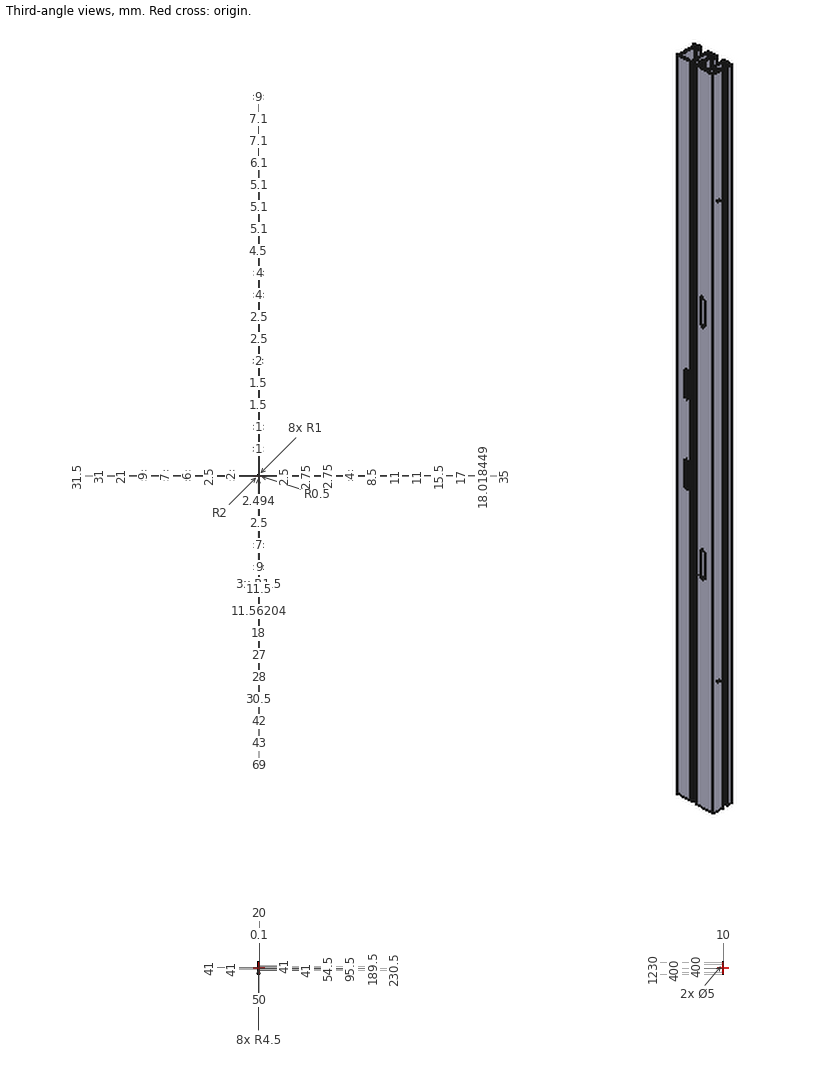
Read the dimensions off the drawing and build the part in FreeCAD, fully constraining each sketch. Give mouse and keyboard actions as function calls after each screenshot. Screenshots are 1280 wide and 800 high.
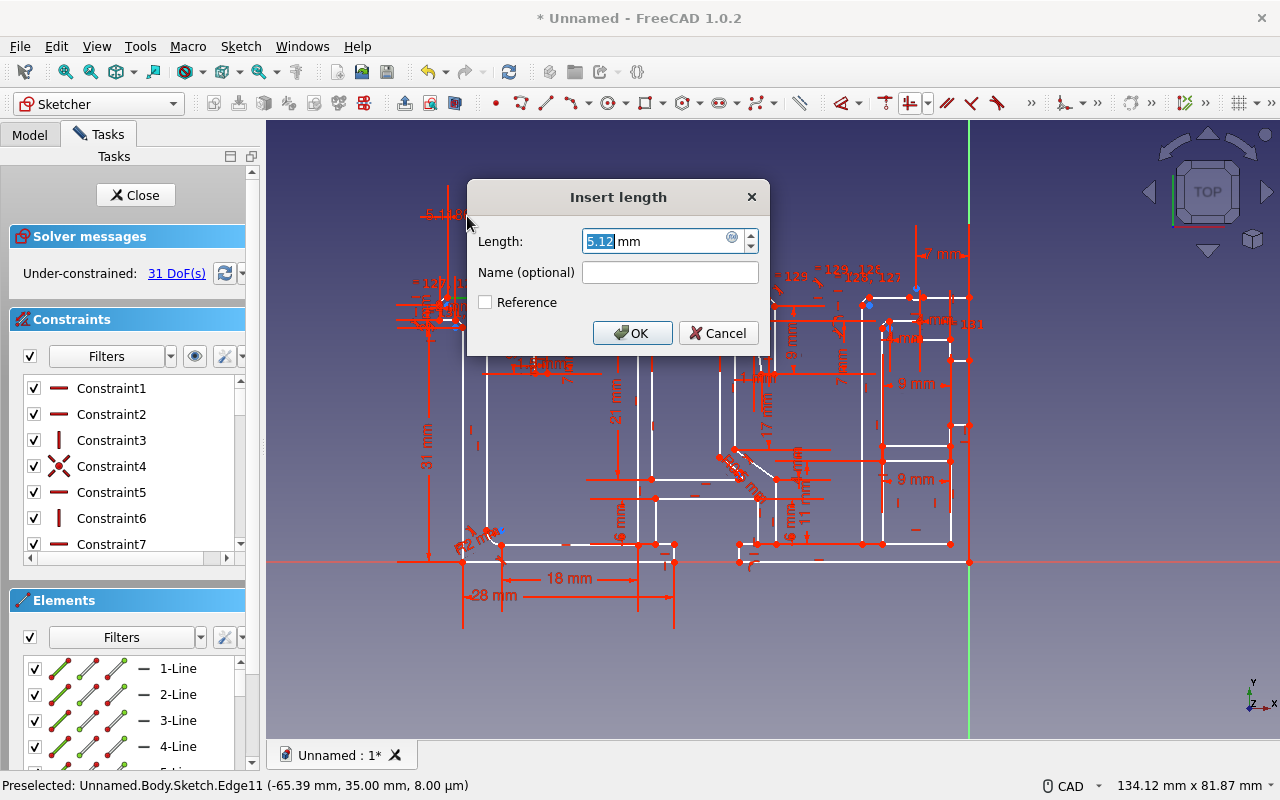
text(5.1)
key(Return)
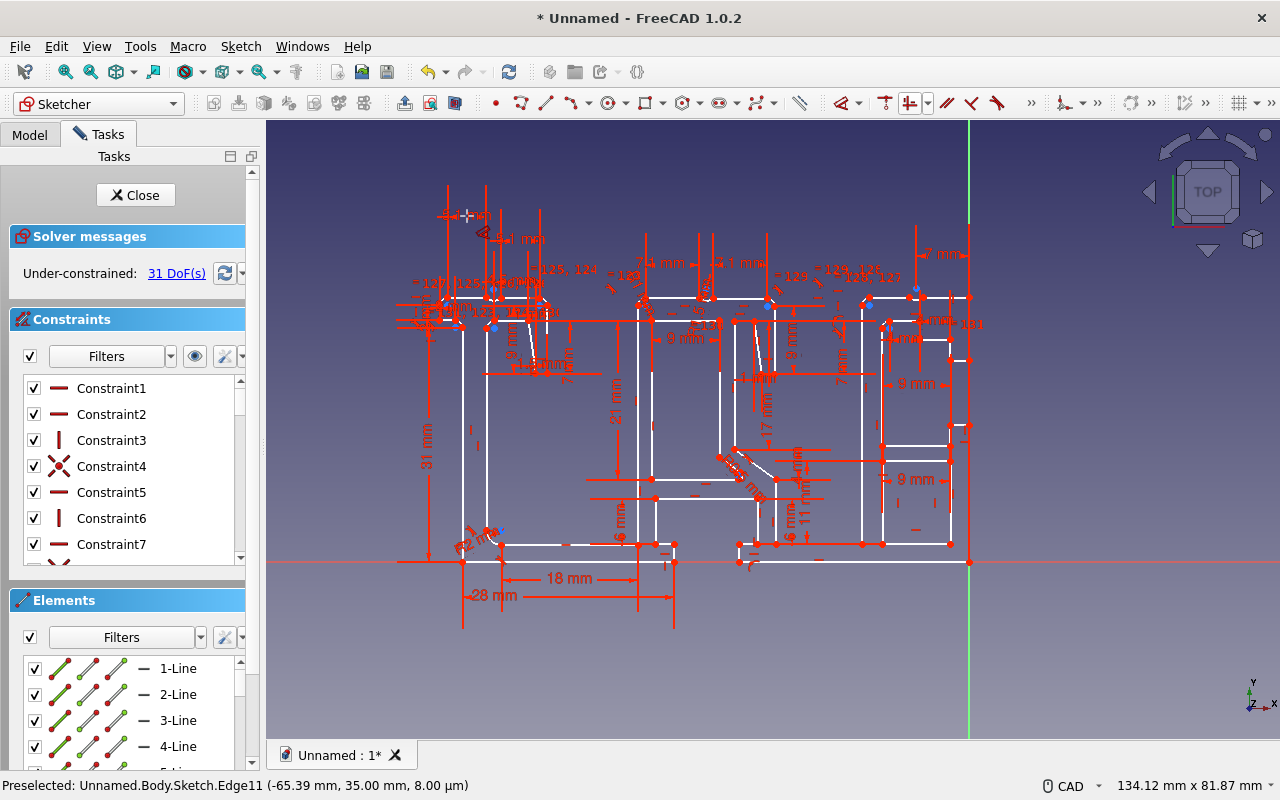
scroll(674, 553, up, 4)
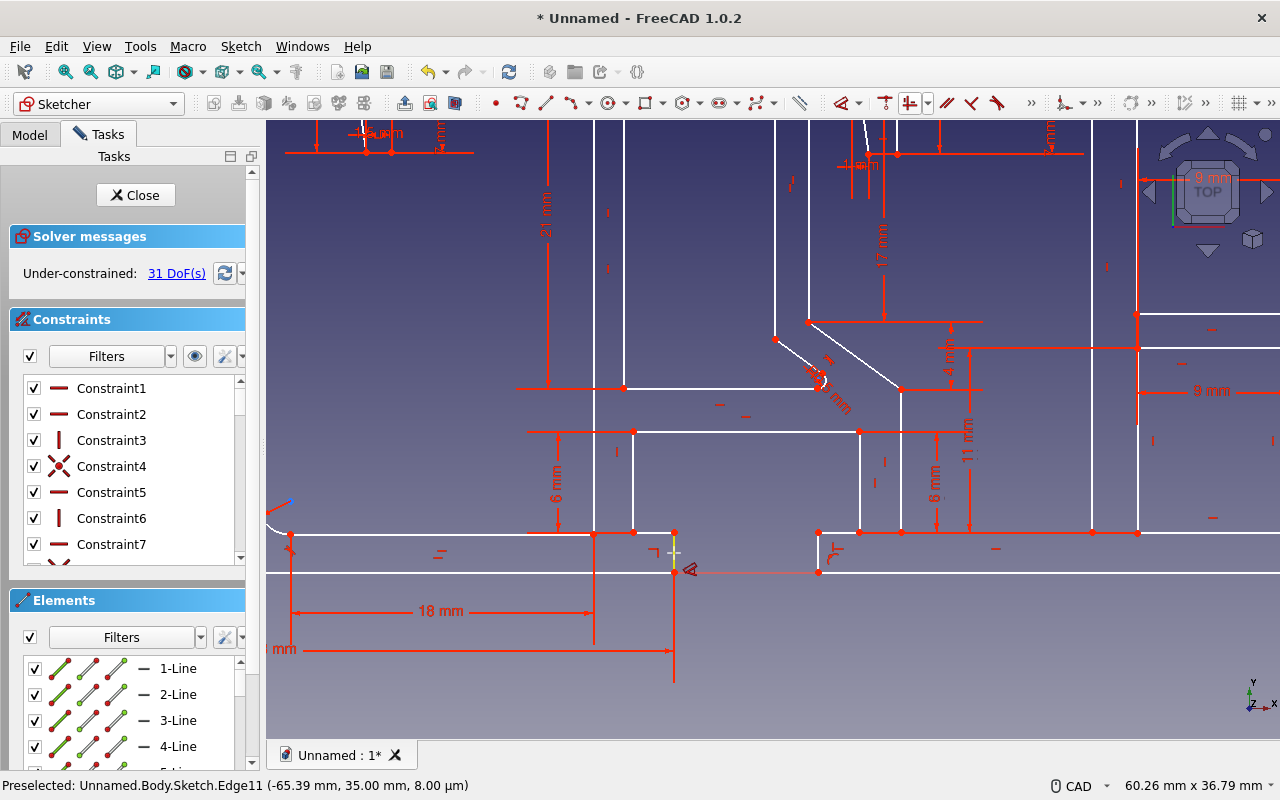
click(674, 553)
click(640, 553)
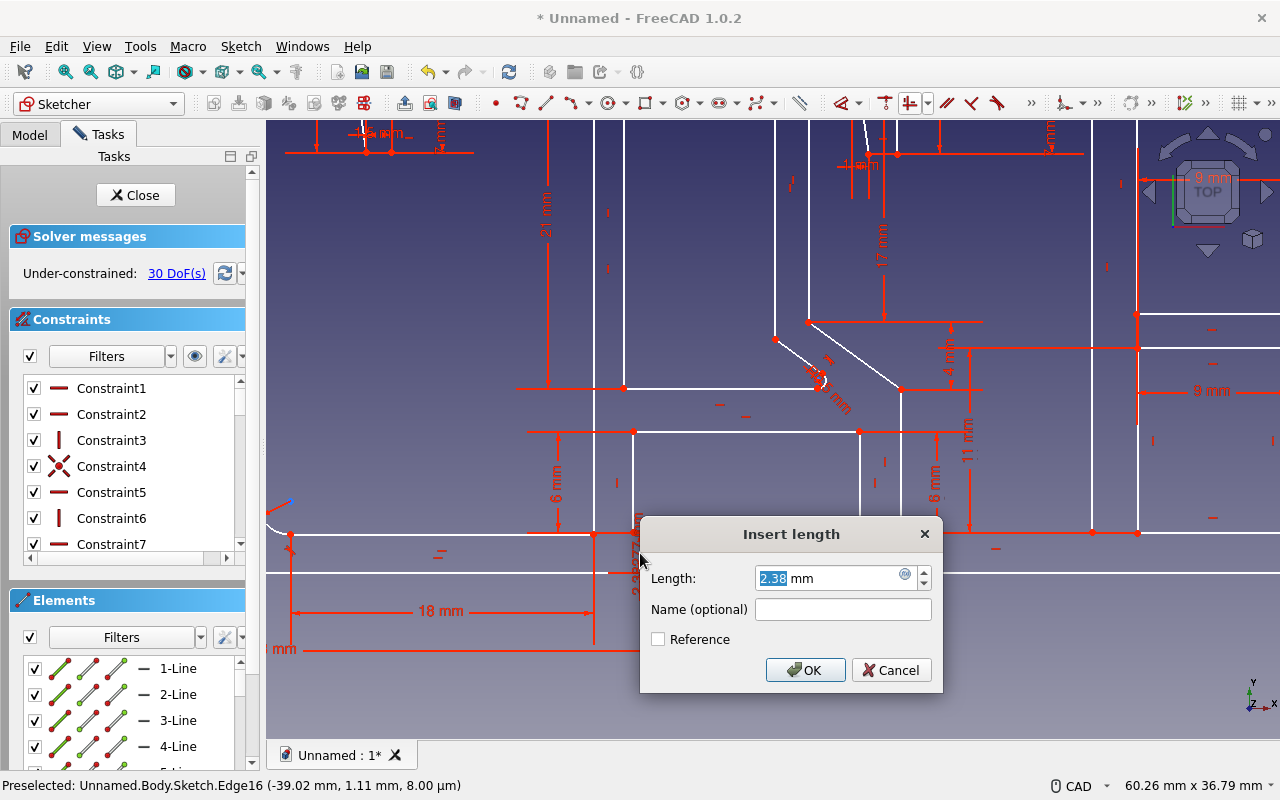
text(2.5)
key(Return)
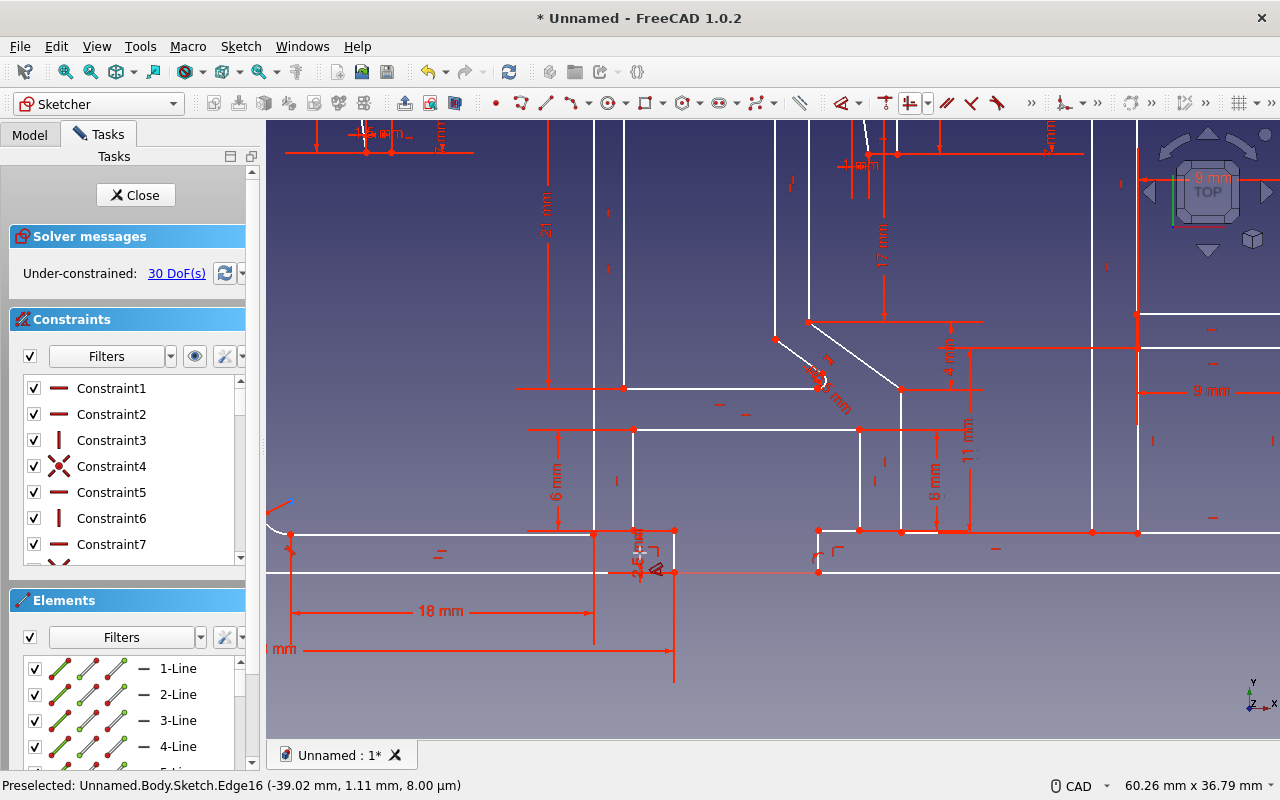
click(662, 531)
click(654, 497)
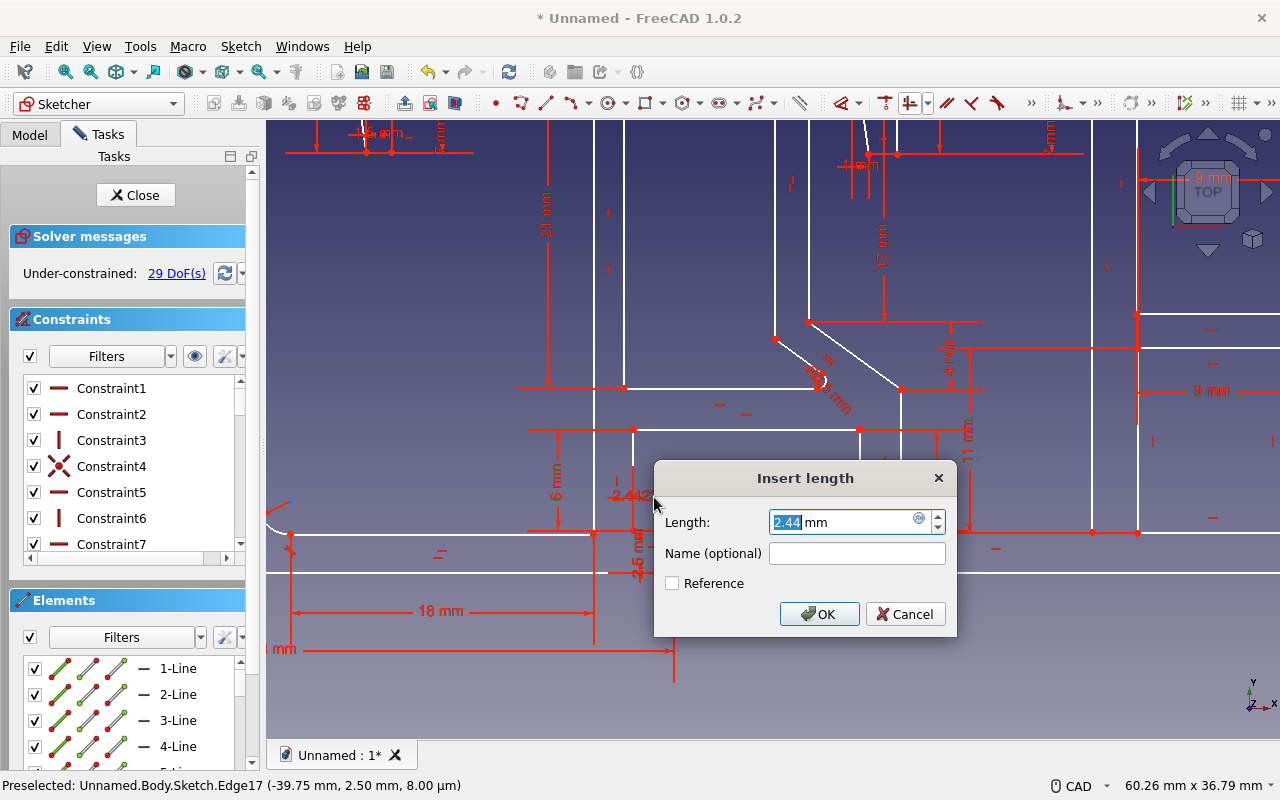
text(2.5)
key(Return)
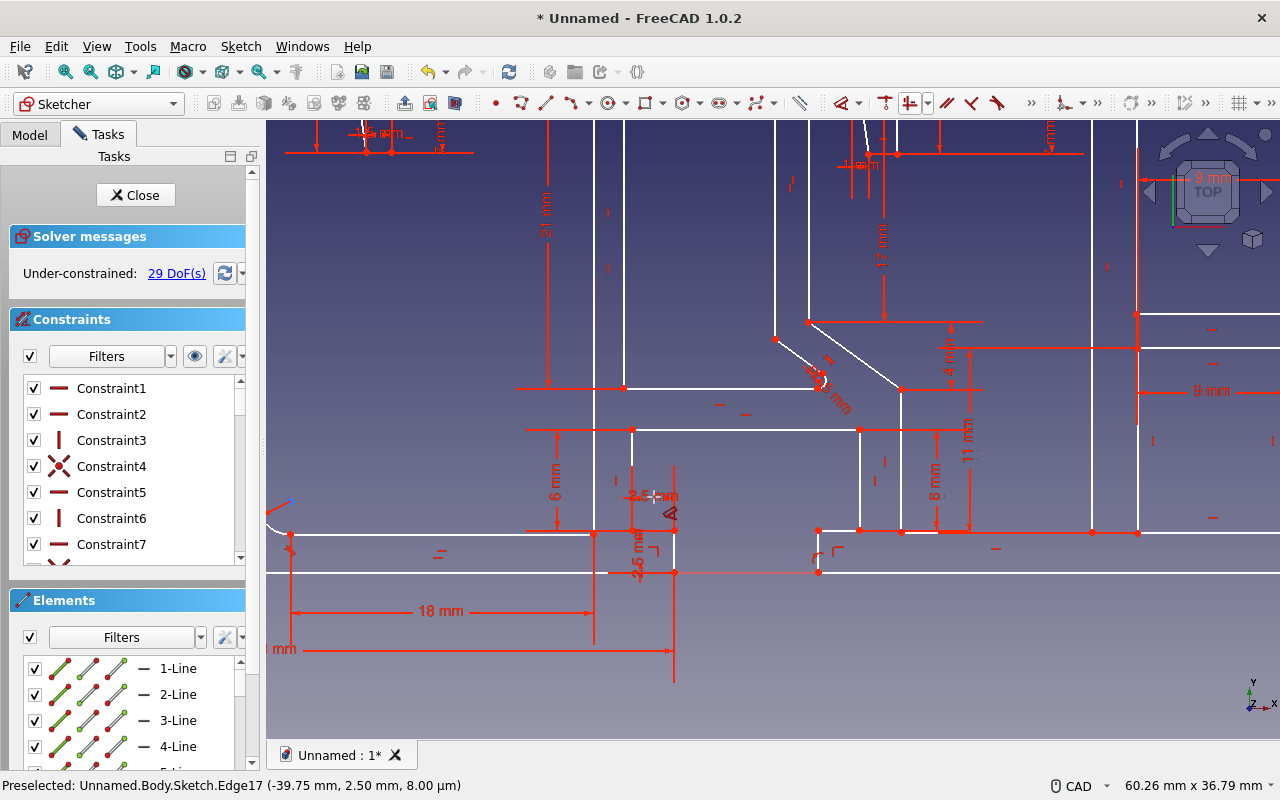
scroll(674, 553, down, 4)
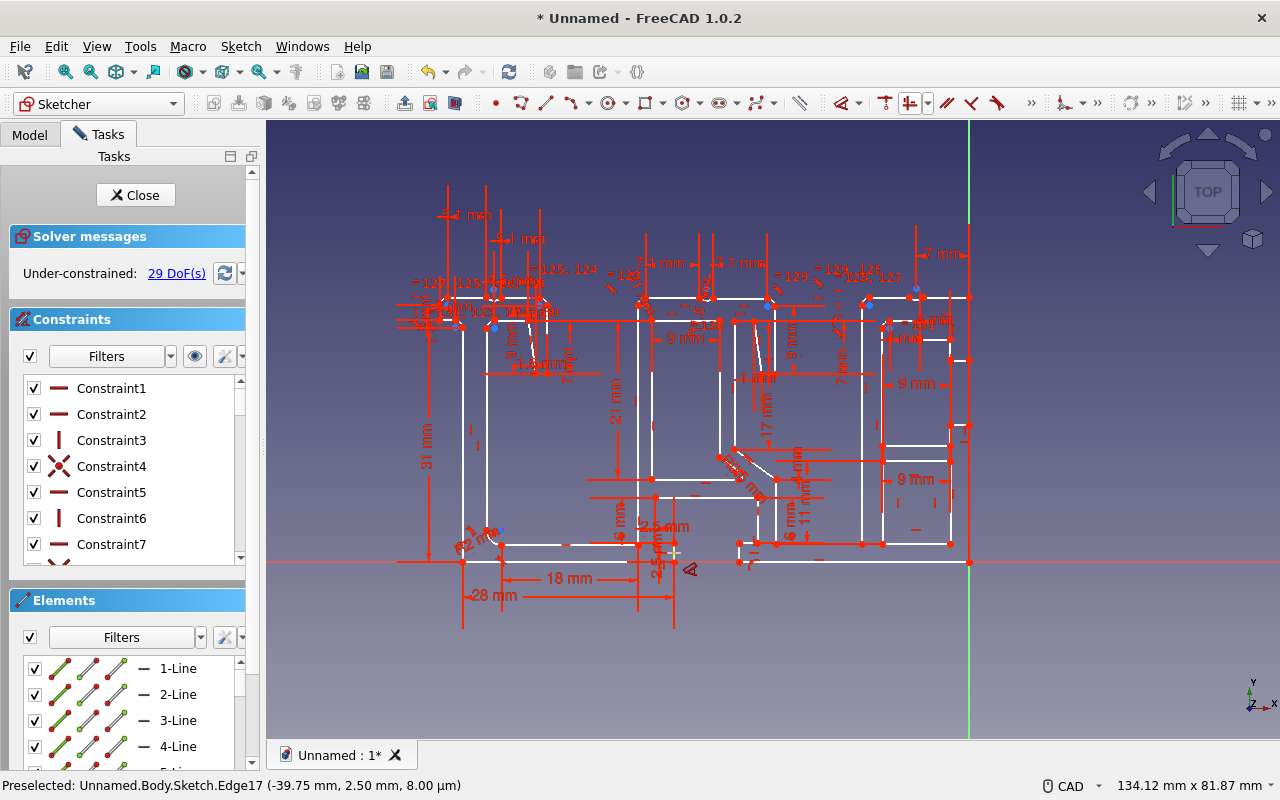
scroll(964, 425, up, 5)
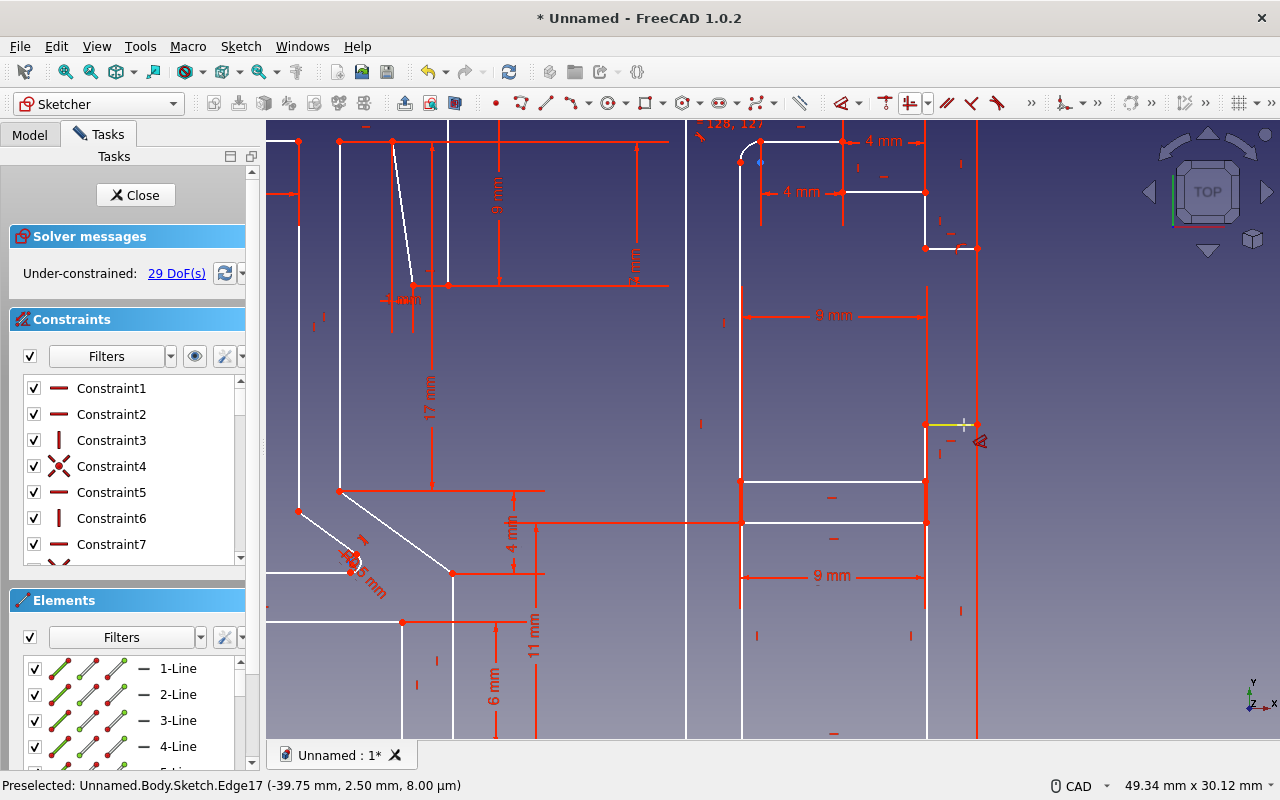
click(962, 425)
click(951, 391)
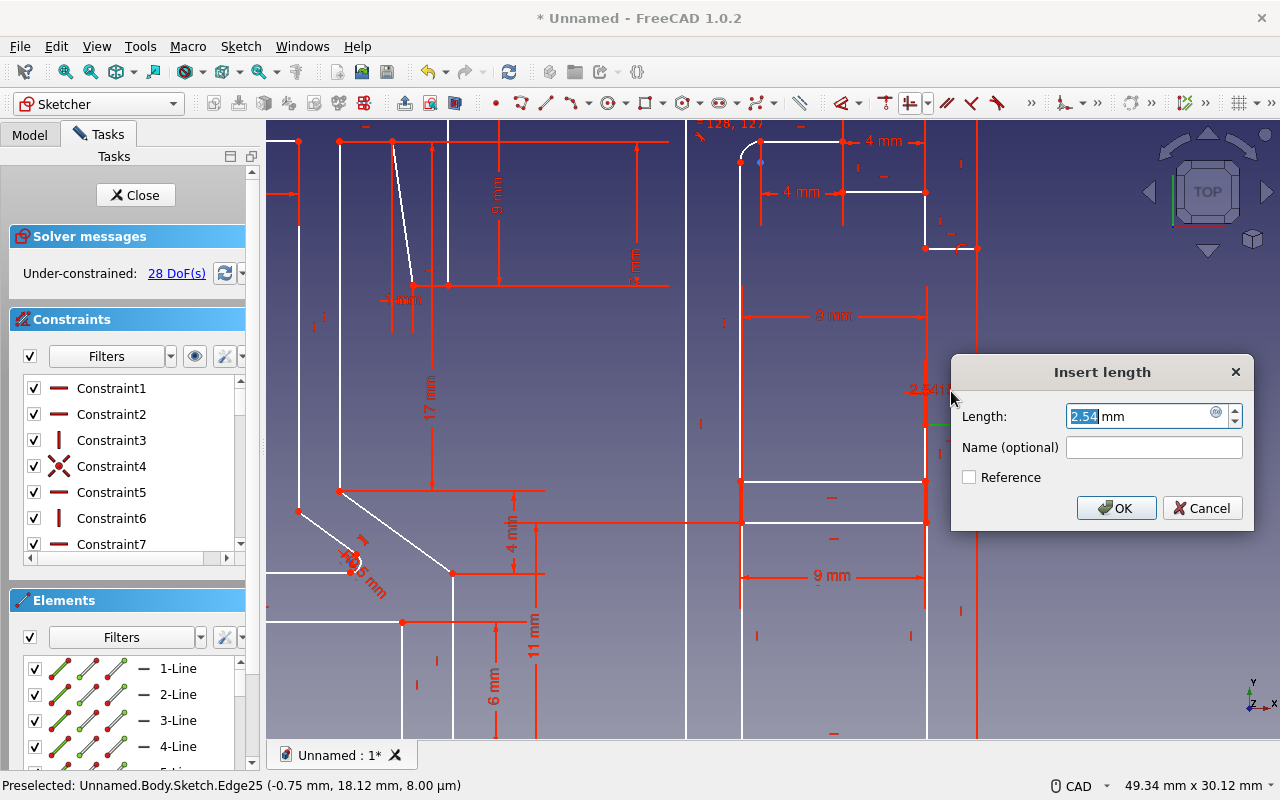
text(2.5)
key(Return)